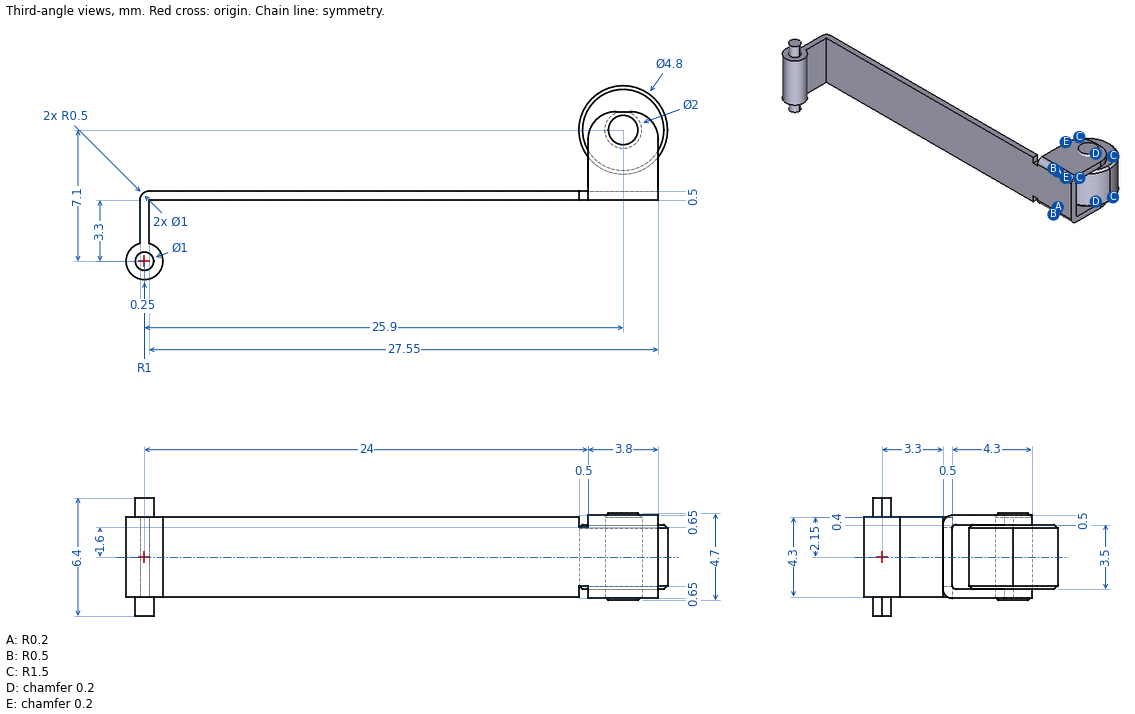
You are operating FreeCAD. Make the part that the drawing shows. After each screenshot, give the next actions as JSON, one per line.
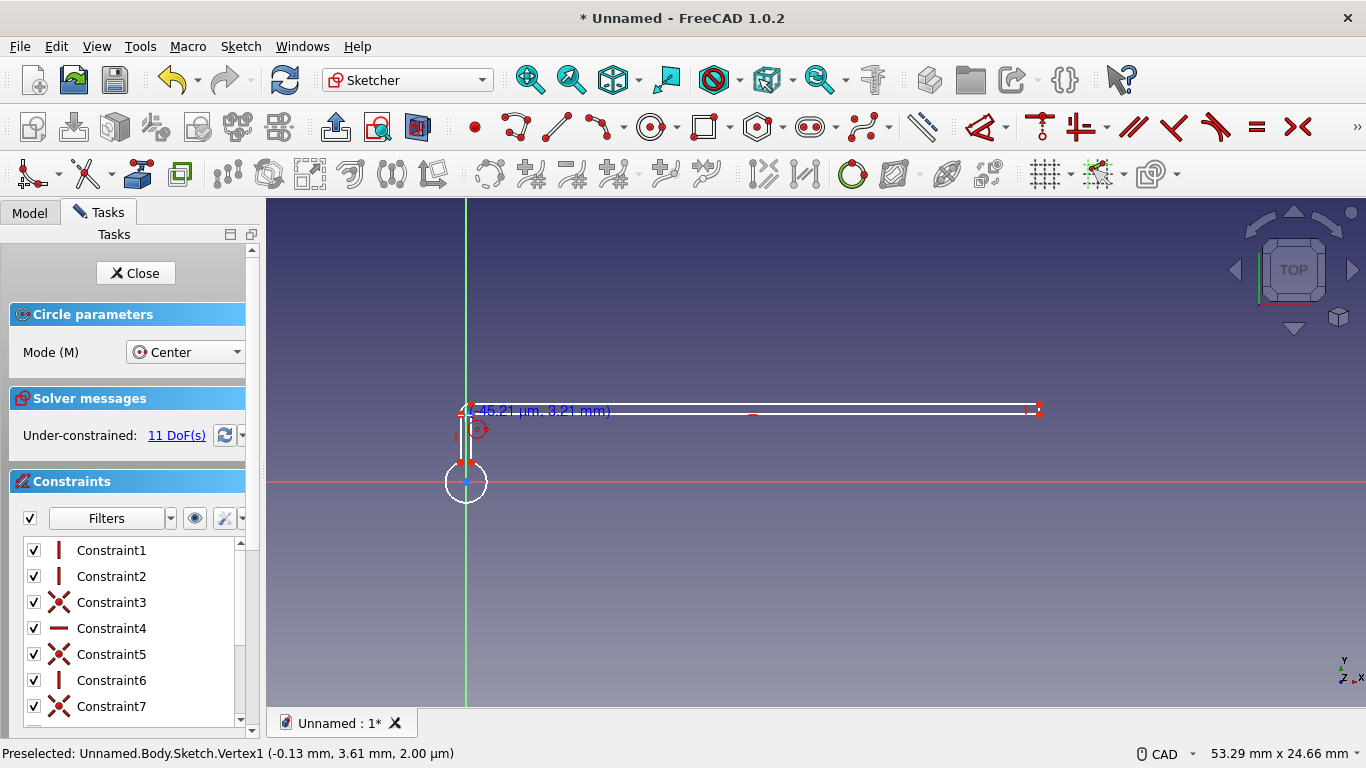
{"action": "scroll", "coordinate": [466, 482], "scroll_direction": "up", "scroll_amount": 4}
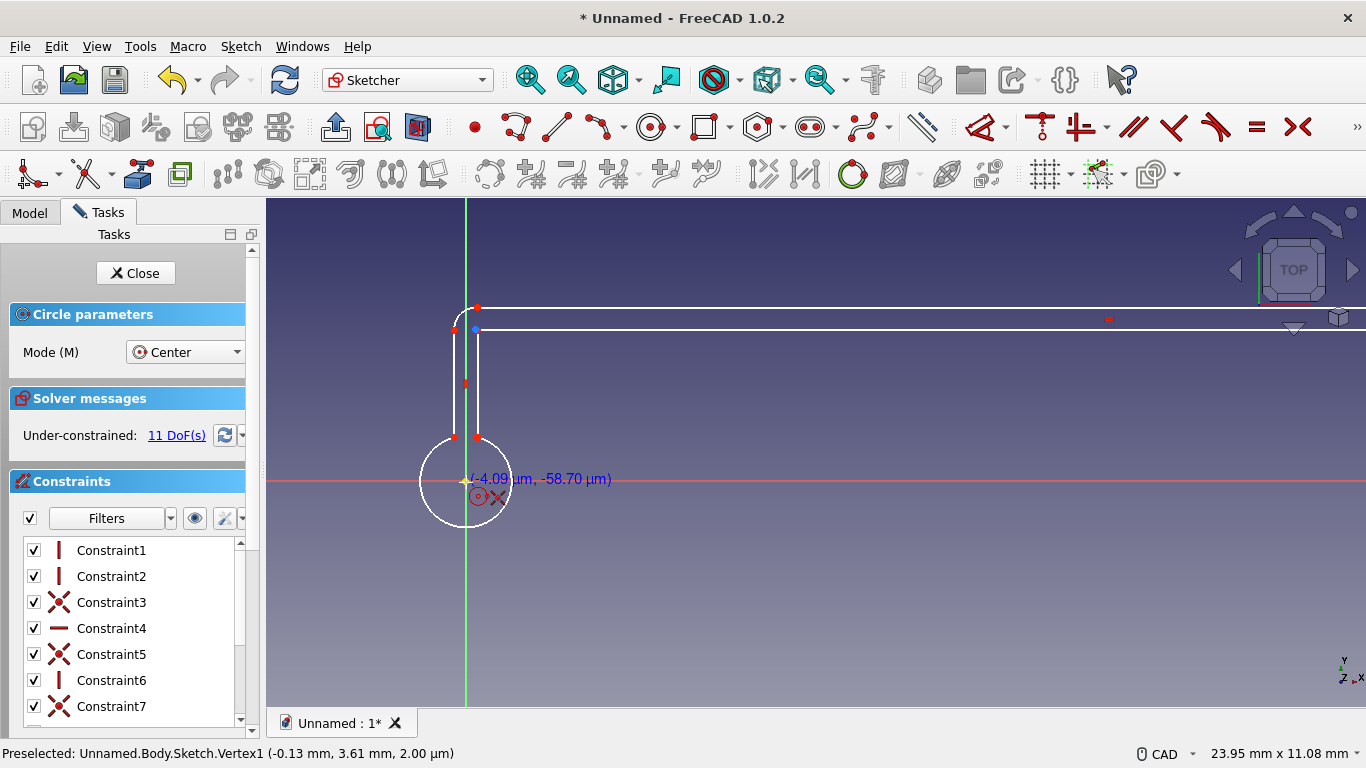
{"action": "left_click", "coordinate": [466, 481]}
{"action": "mouse_move", "coordinate": [482, 465]}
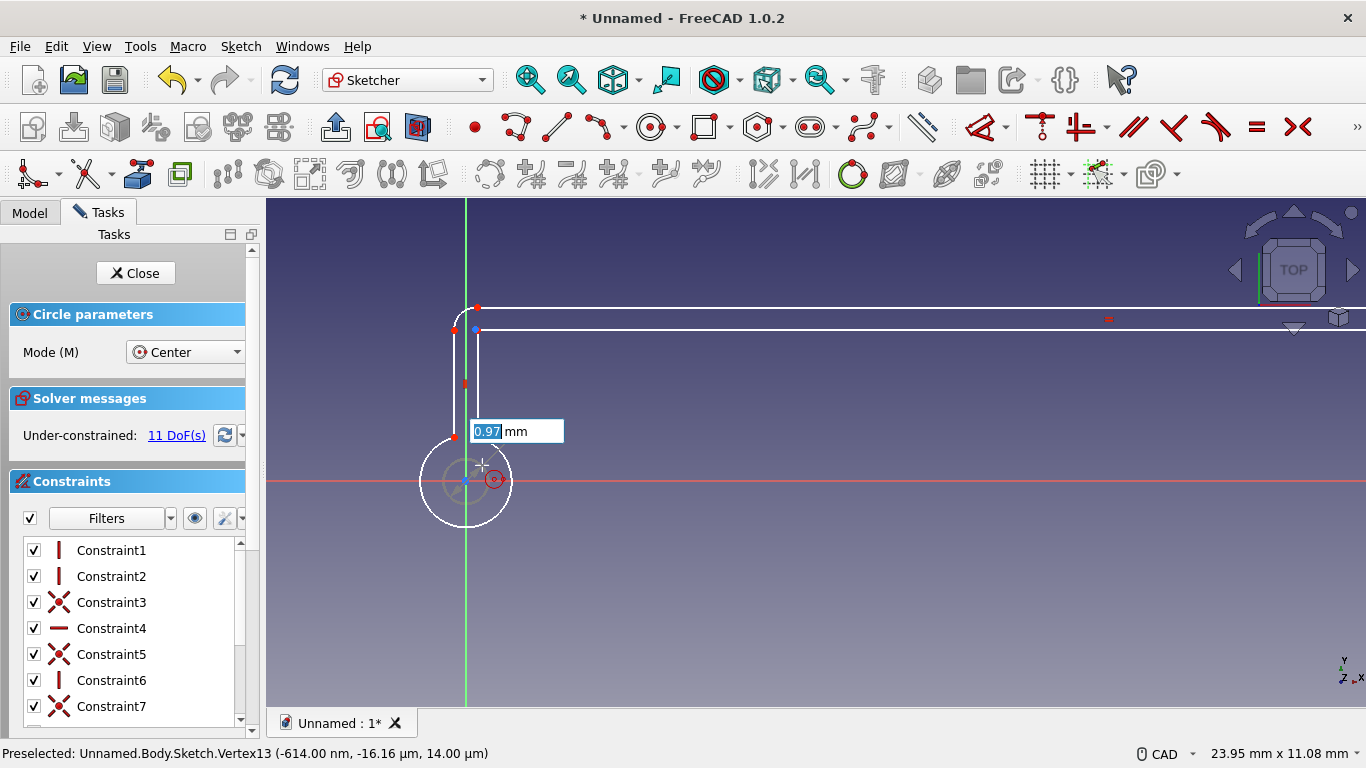
{"action": "type", "text": "1"}
{"action": "key", "text": "Return"}
{"action": "key", "text": "Escape"}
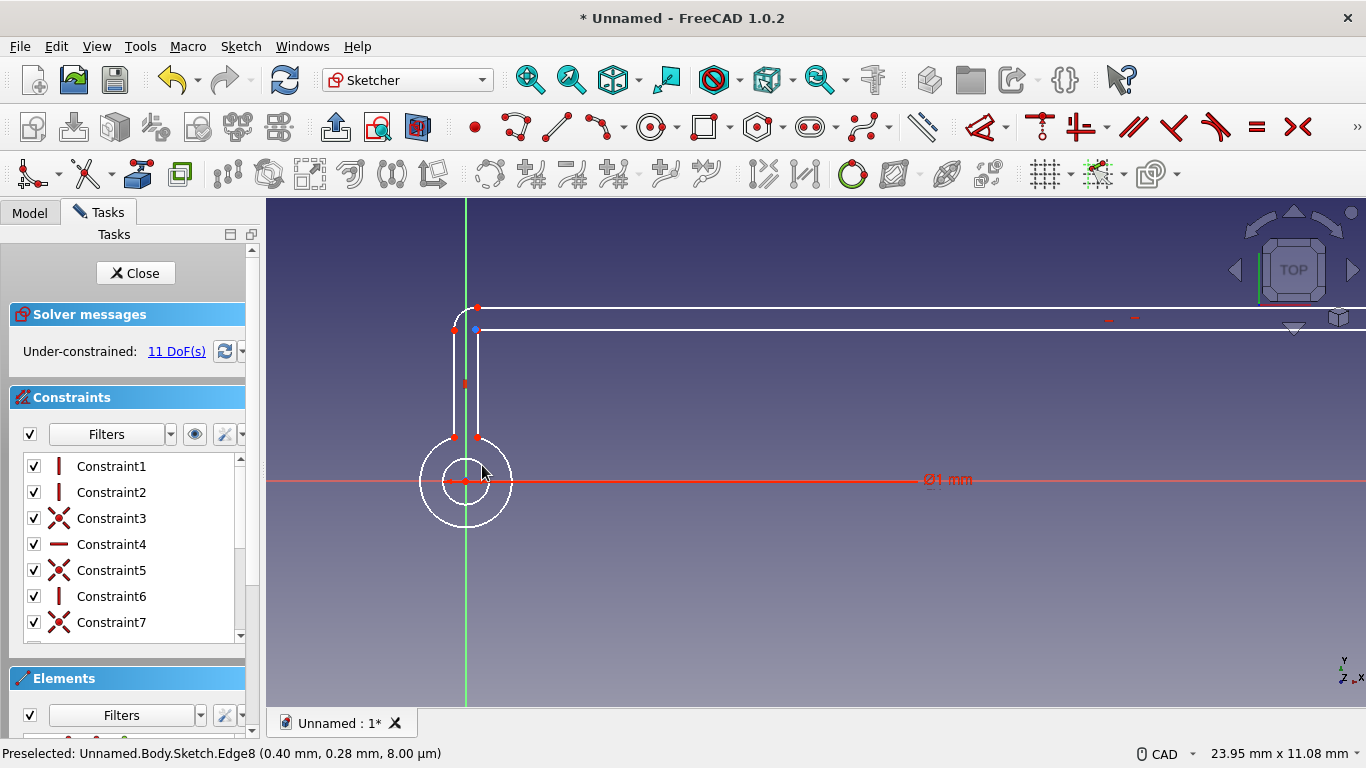
{"action": "left_click", "coordinate": [454, 362]}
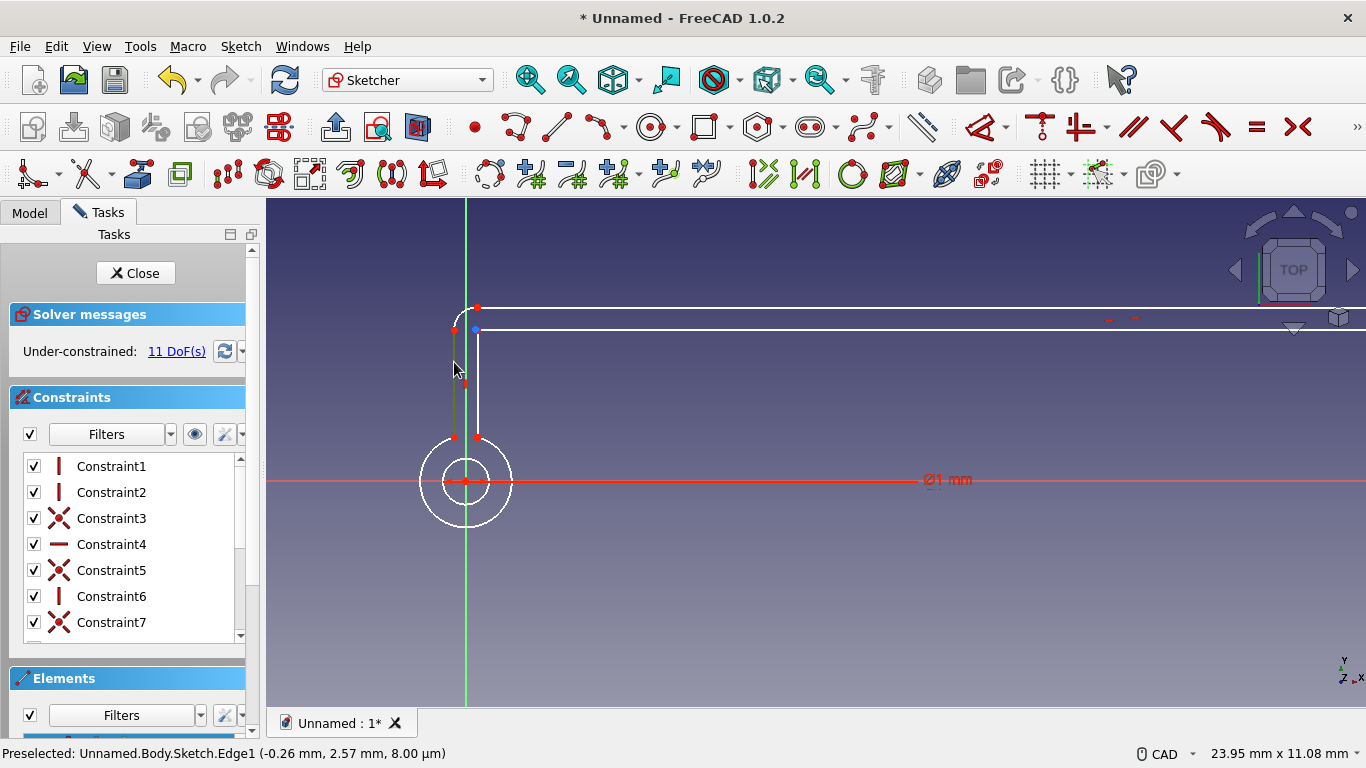
{"action": "scroll", "coordinate": [467, 310], "scroll_direction": "up", "scroll_amount": 2}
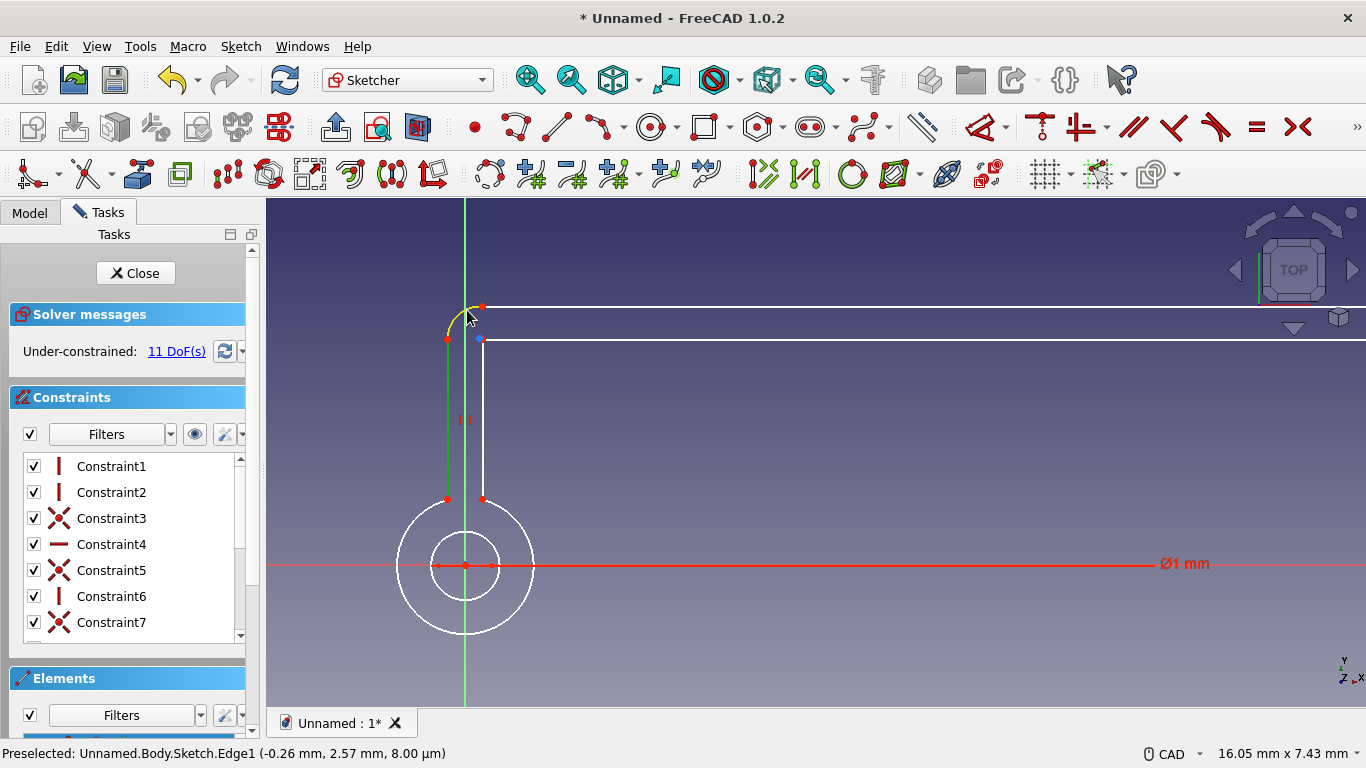
{"action": "left_click", "coordinate": [466, 310]}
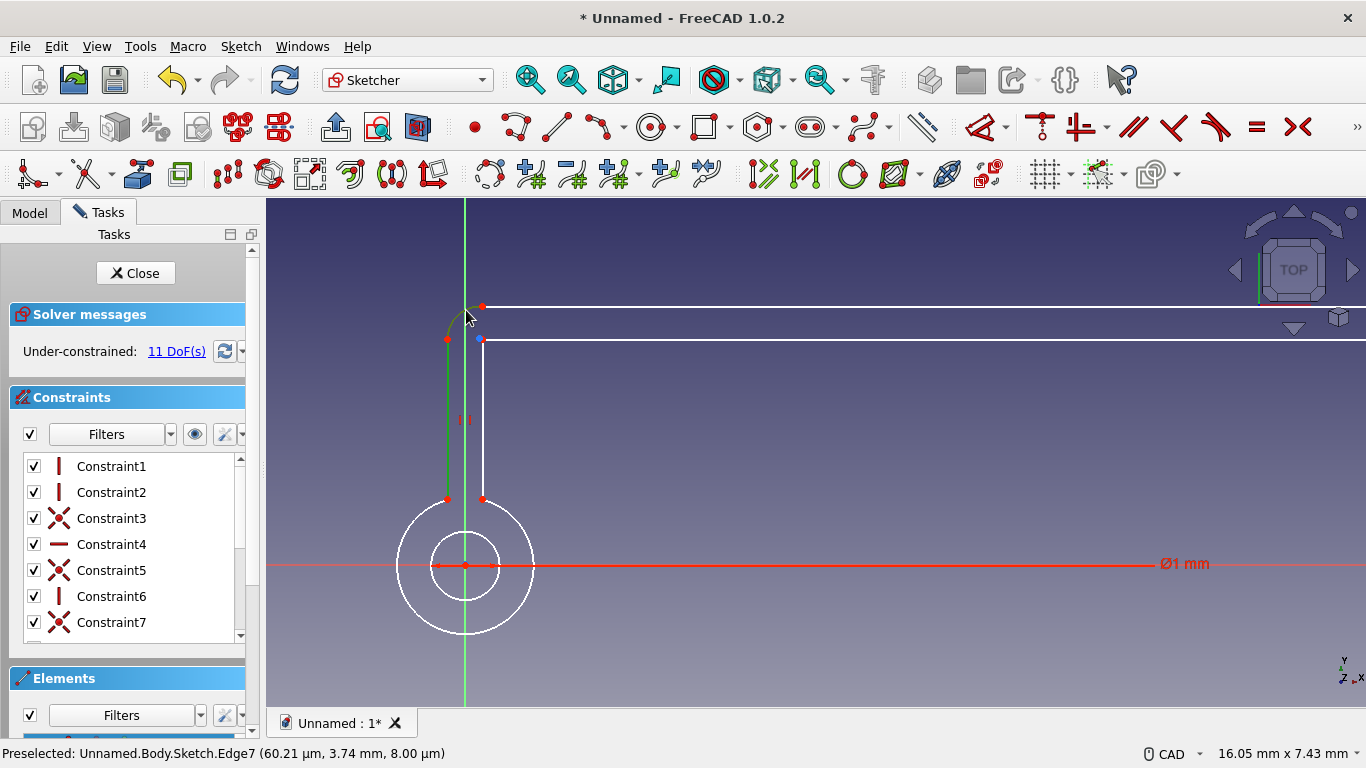
{"action": "left_click", "coordinate": [1216, 128]}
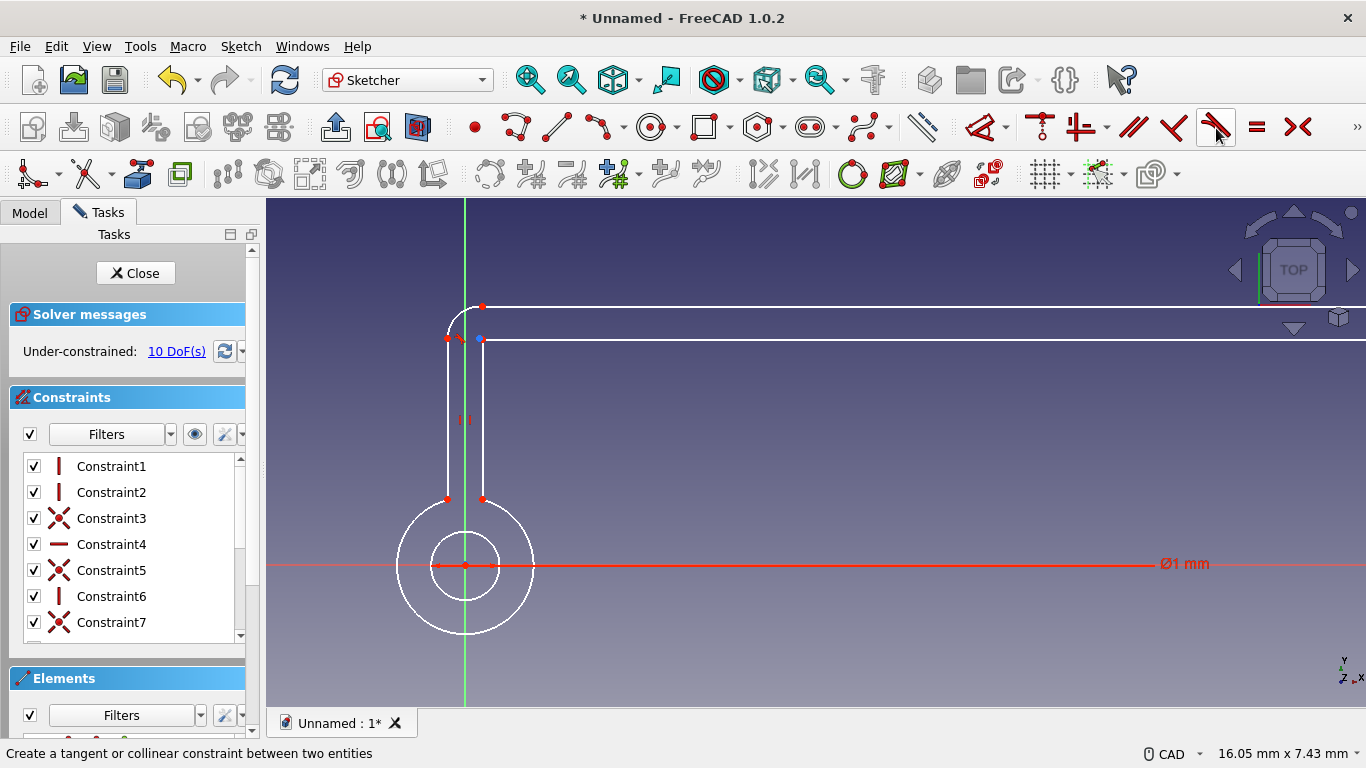
{"action": "left_click", "coordinate": [1048, 307]}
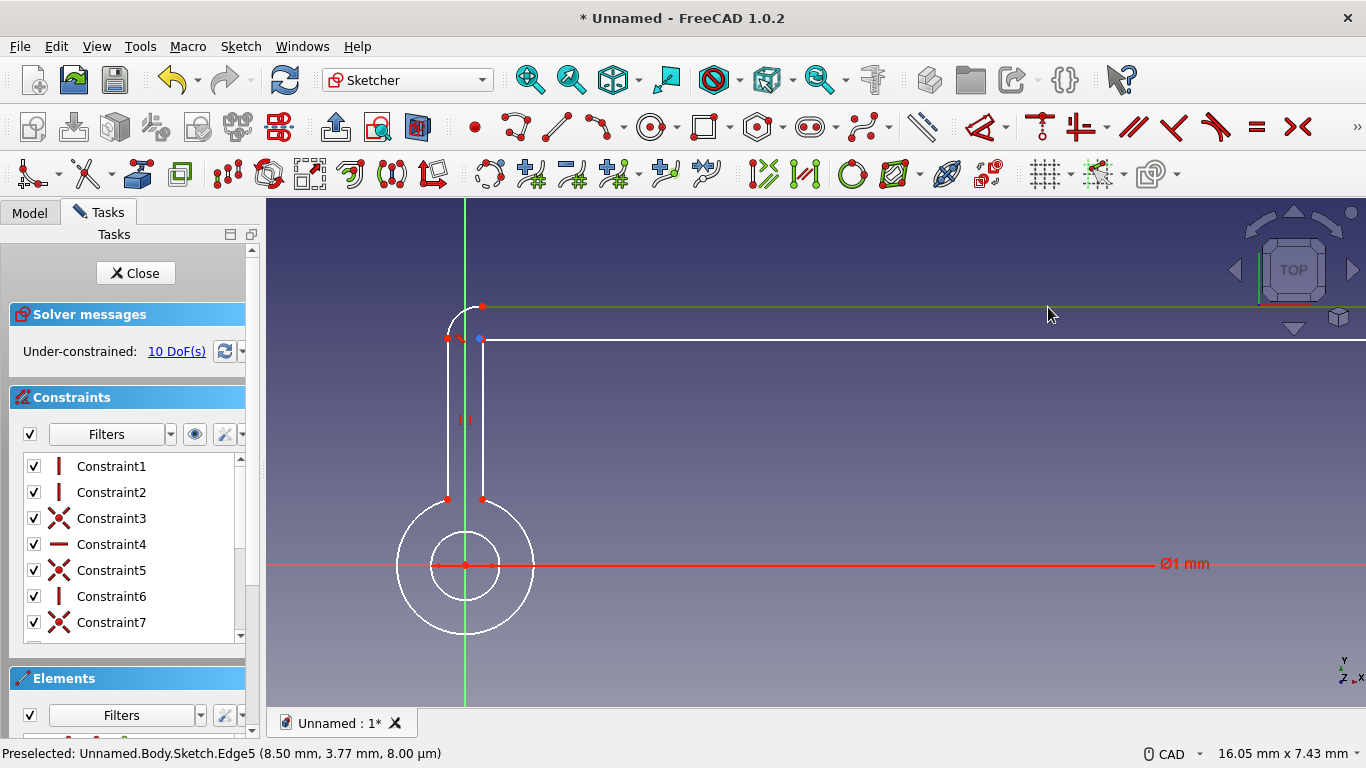
{"action": "left_click", "coordinate": [467, 309]}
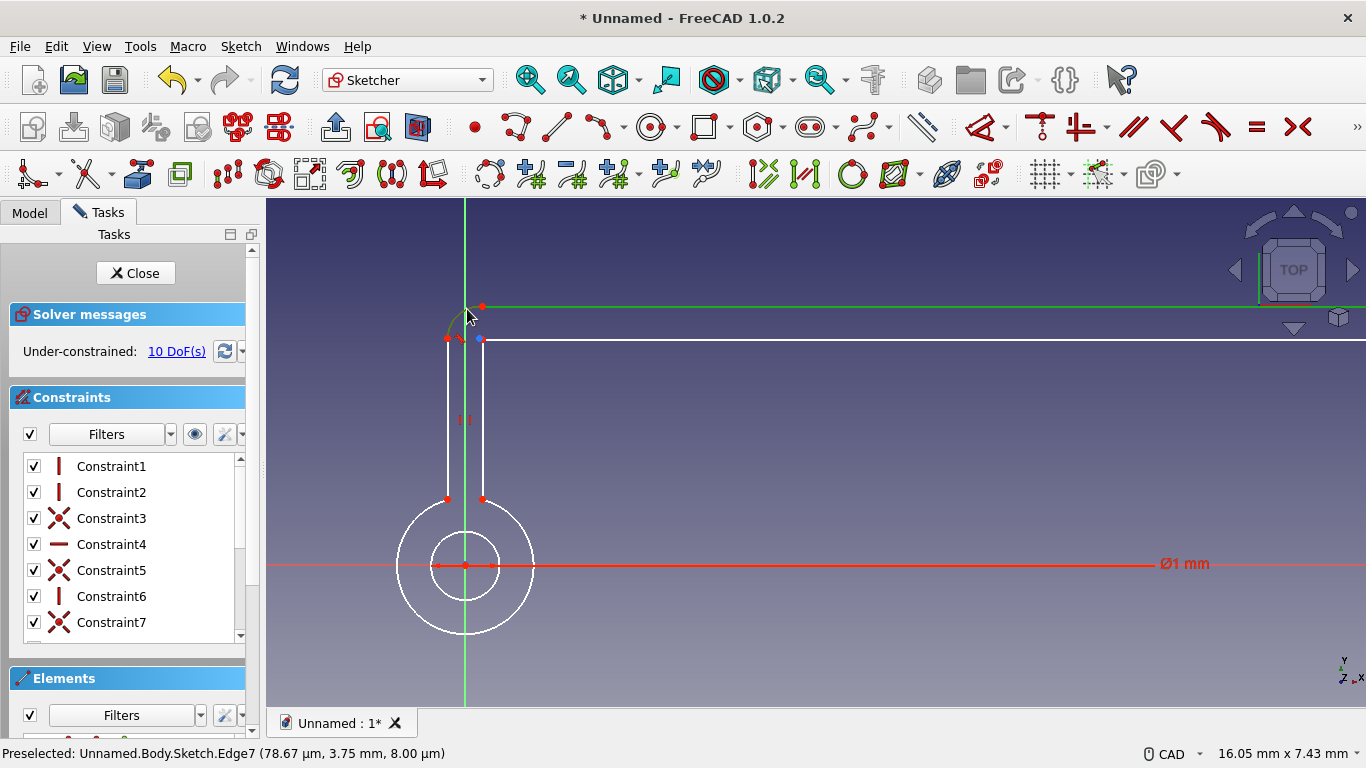
{"action": "key", "text": "t"}